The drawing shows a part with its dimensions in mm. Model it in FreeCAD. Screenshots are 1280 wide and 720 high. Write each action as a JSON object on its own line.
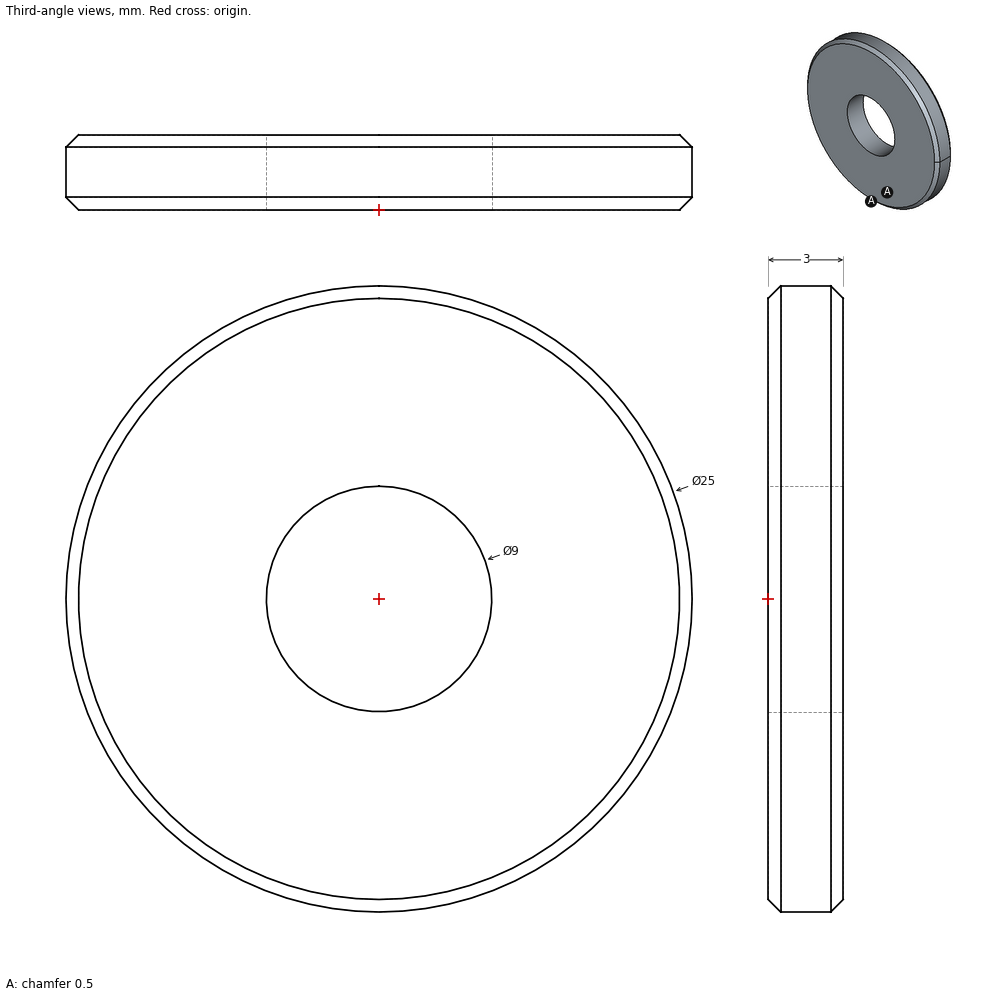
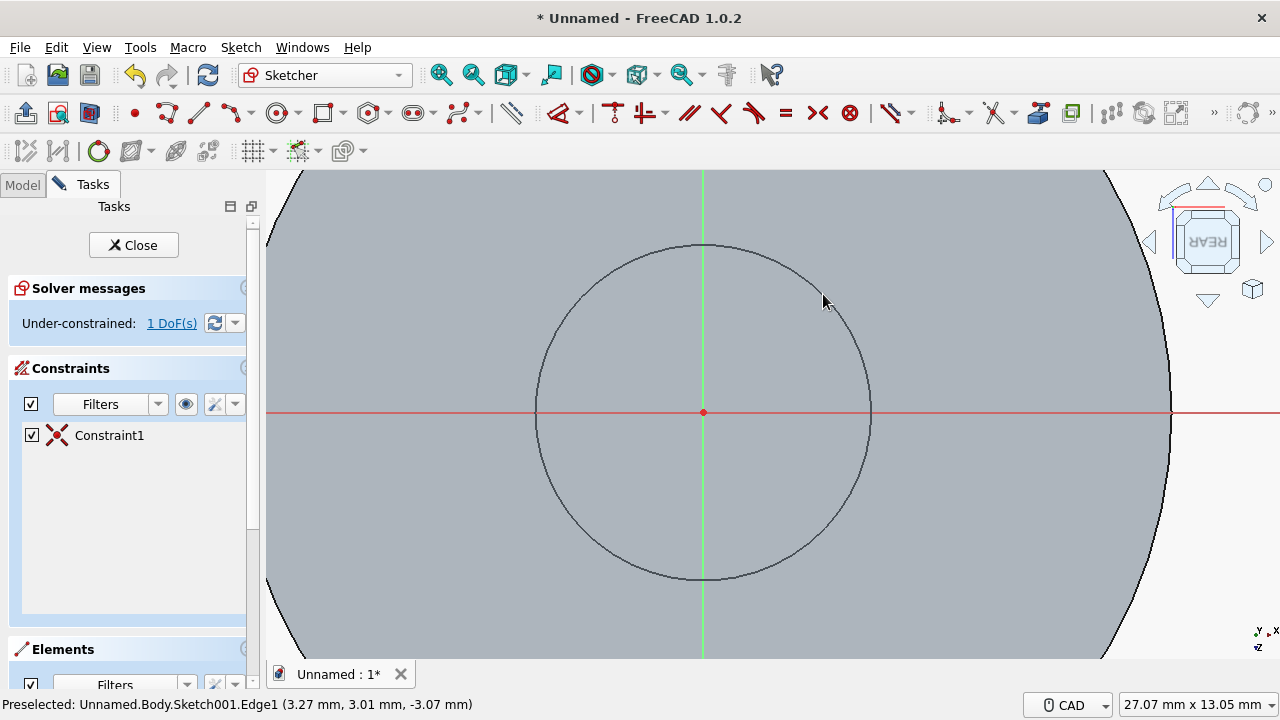
{"action": "left_click", "coordinate": [558, 114]}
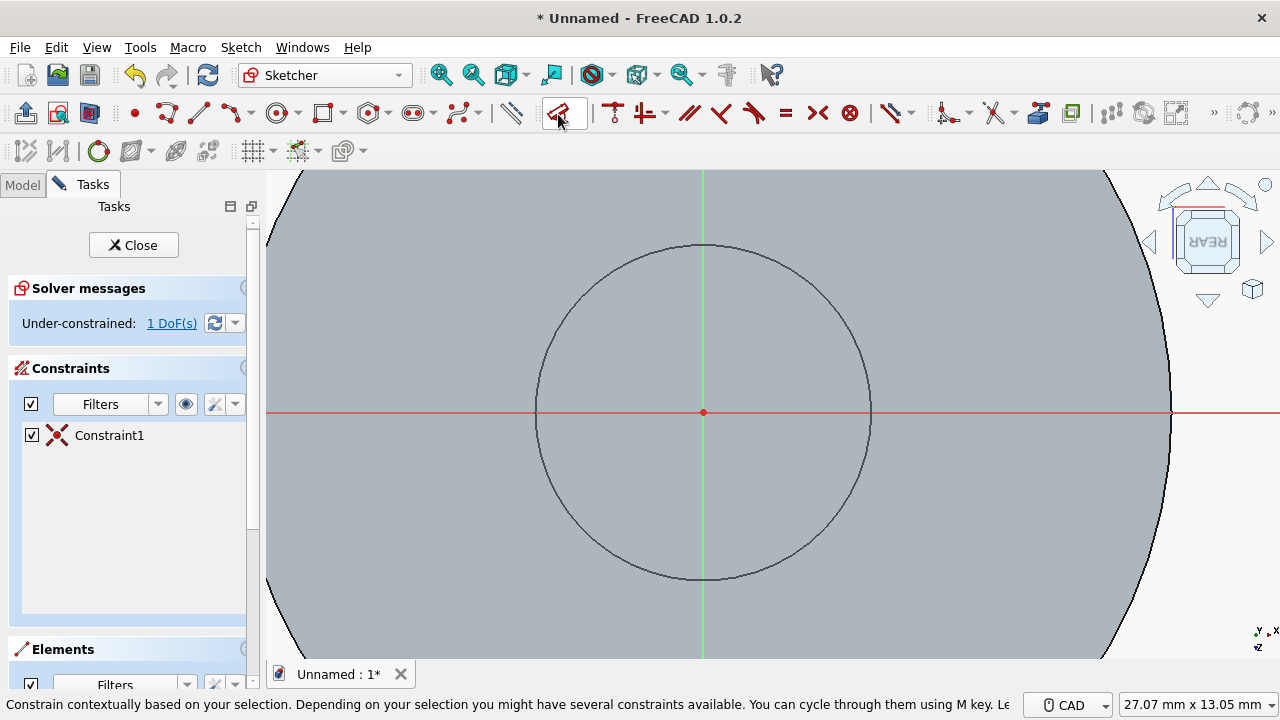
{"action": "left_click", "coordinate": [822, 294]}
{"action": "left_click", "coordinate": [845, 271]}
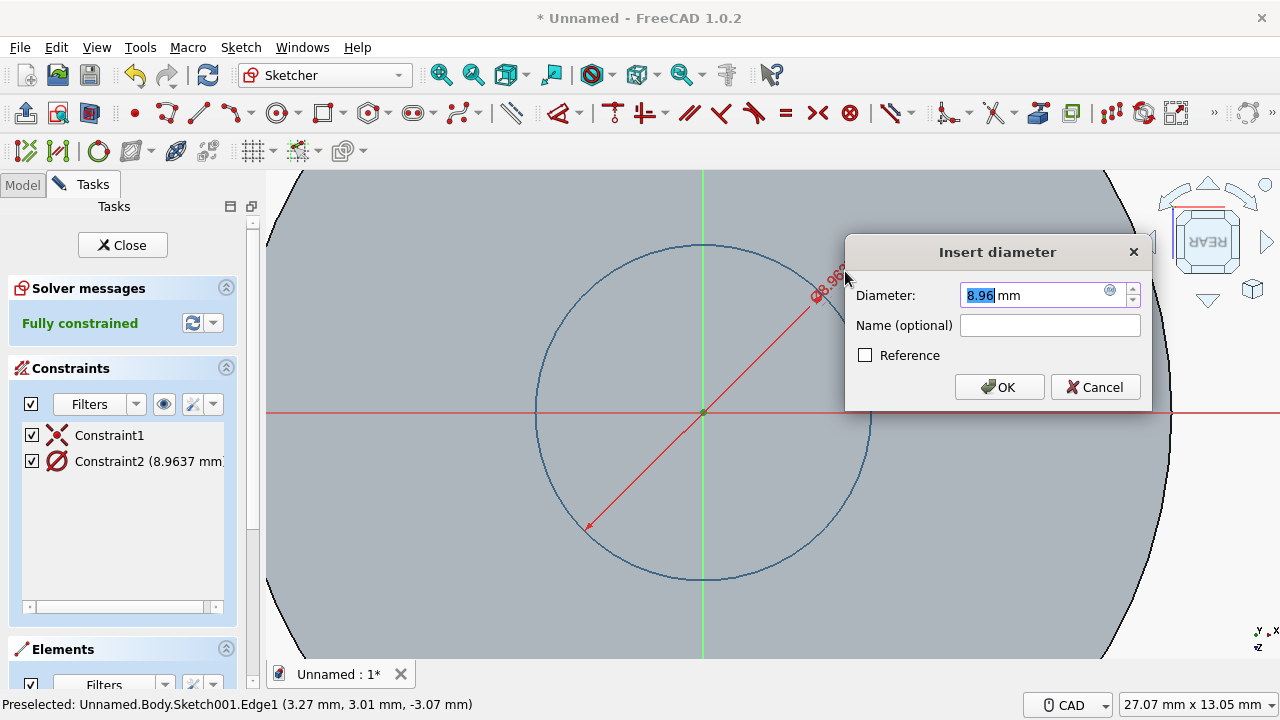
{"action": "type", "text": "9"}
{"action": "key", "text": "Return"}
{"action": "key", "text": "Escape"}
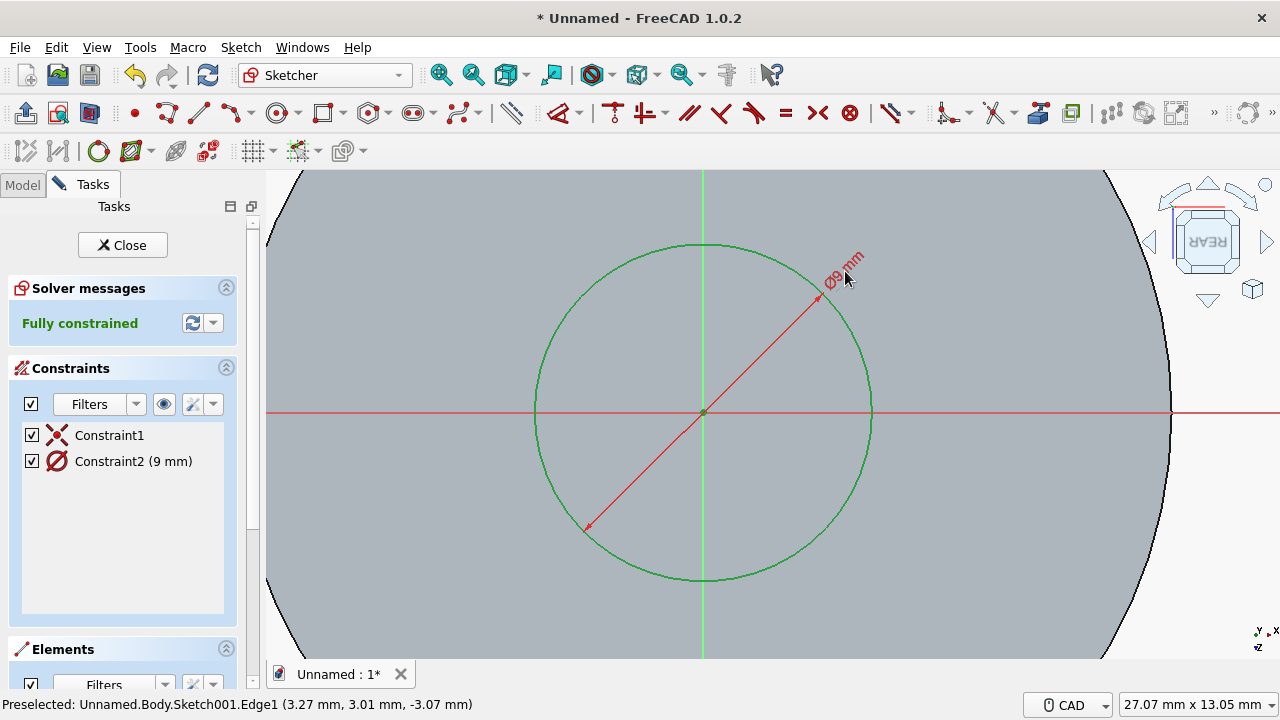
{"action": "left_click", "coordinate": [123, 245]}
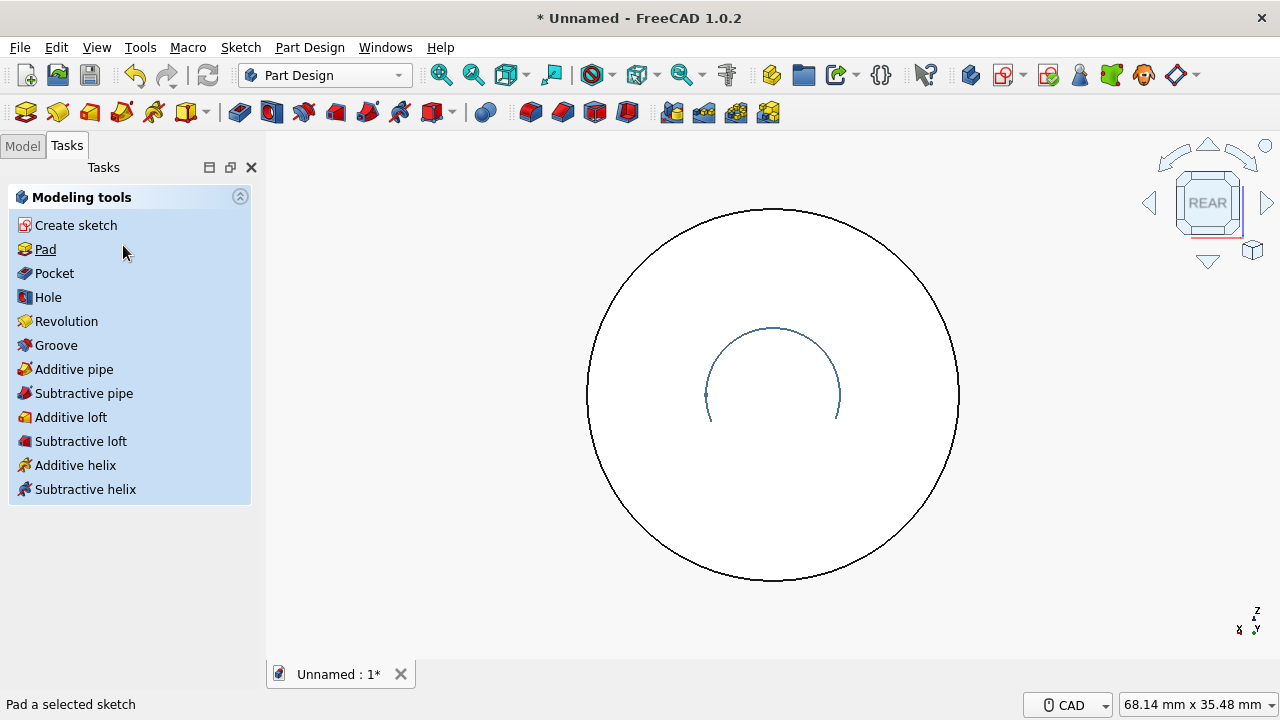
{"action": "left_click", "coordinate": [240, 112]}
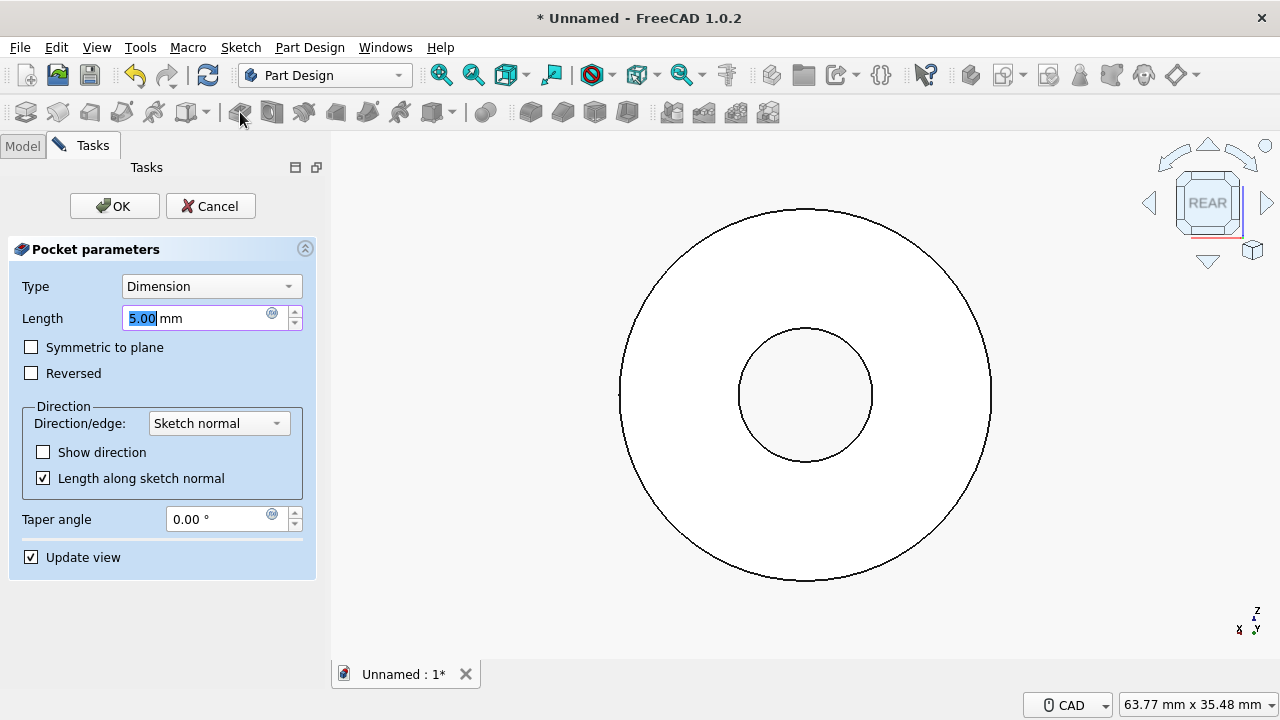
{"action": "left_click", "coordinate": [212, 286]}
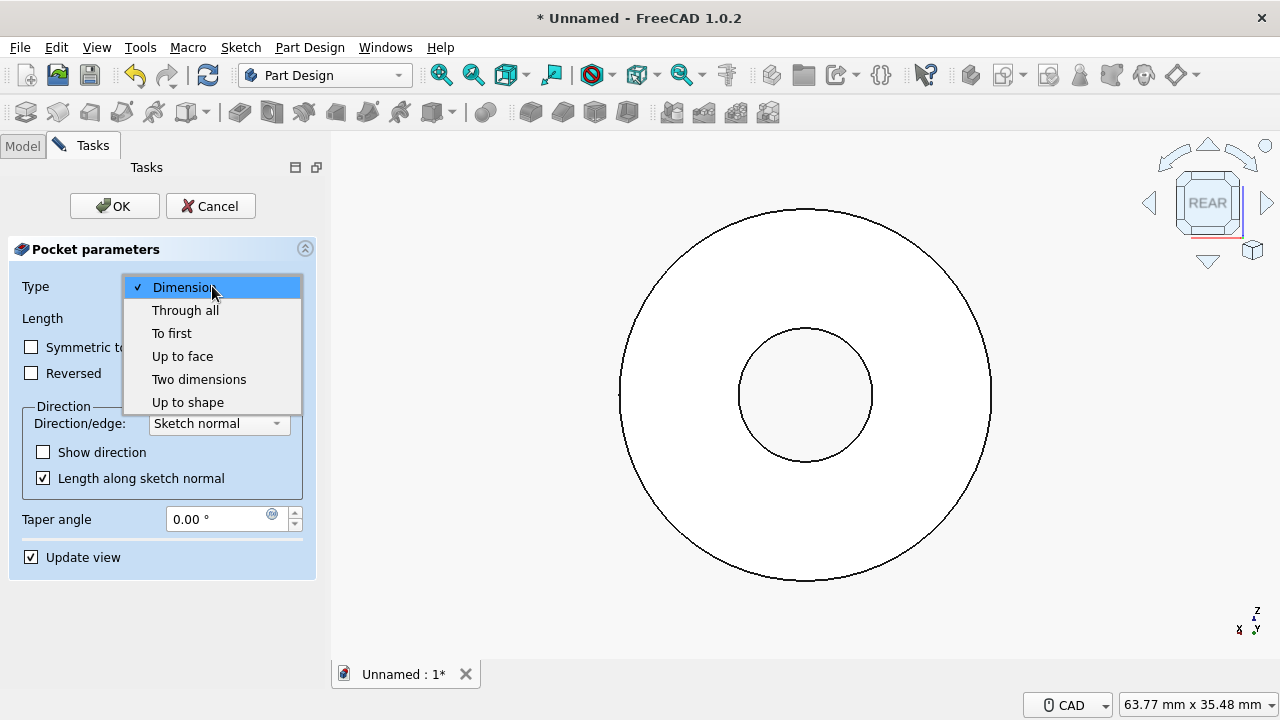
{"action": "left_click", "coordinate": [212, 310]}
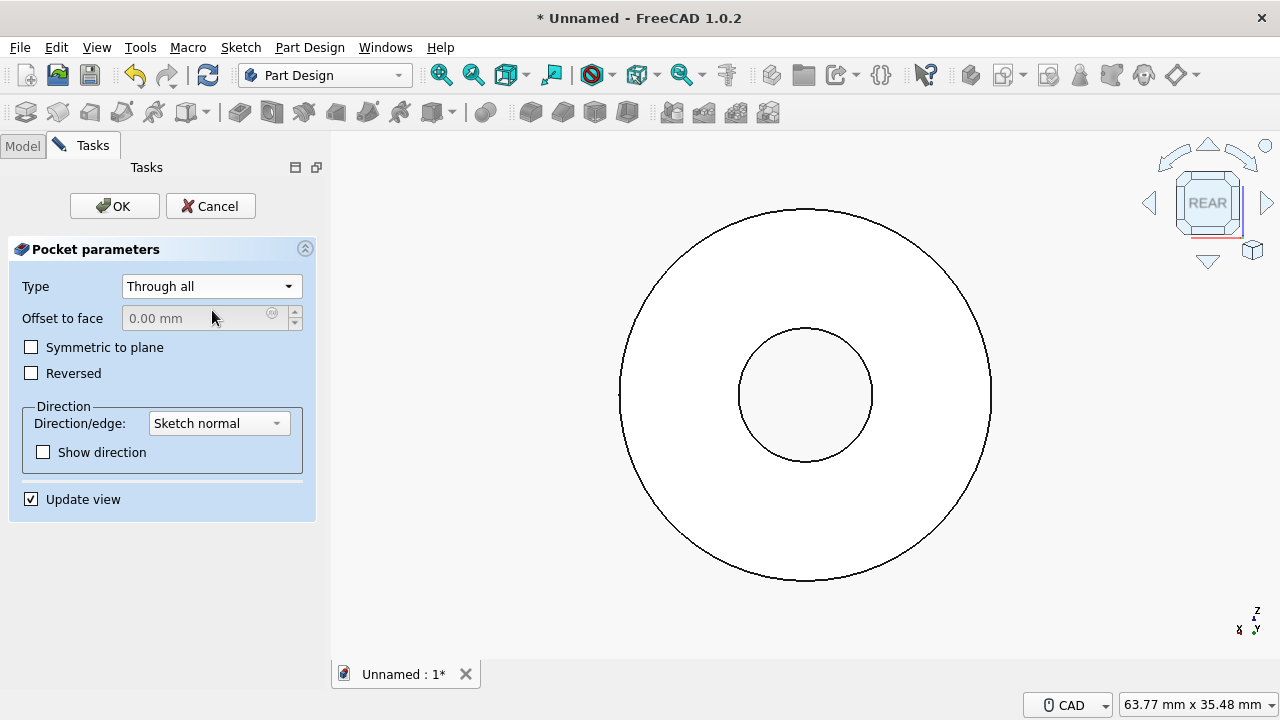
{"action": "left_click", "coordinate": [115, 206]}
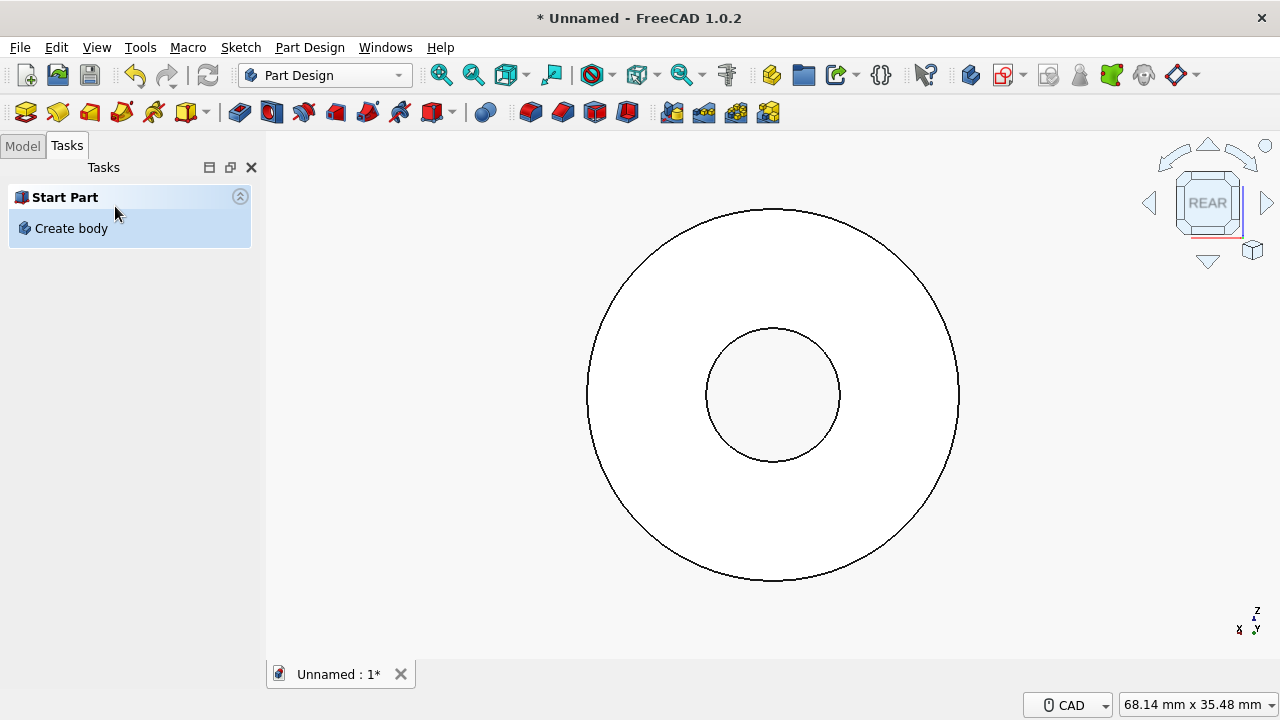
{"action": "left_click", "coordinate": [959, 394]}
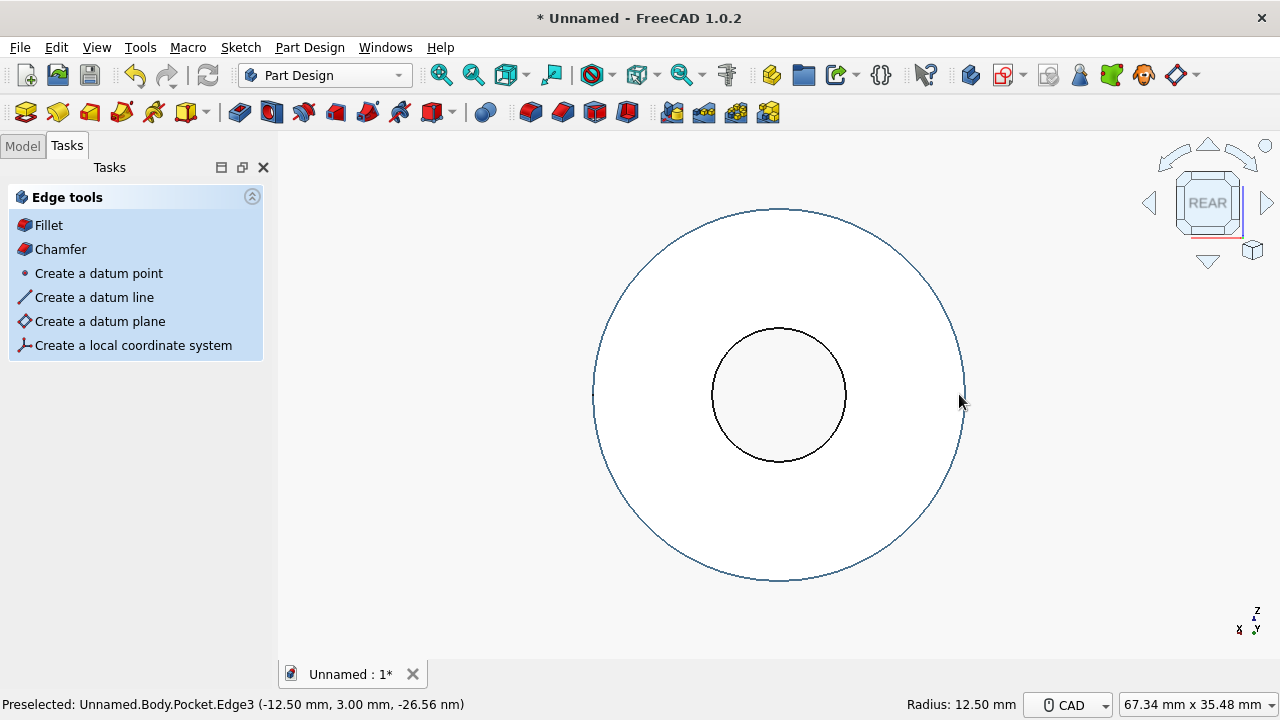
{"action": "key", "text": "0"}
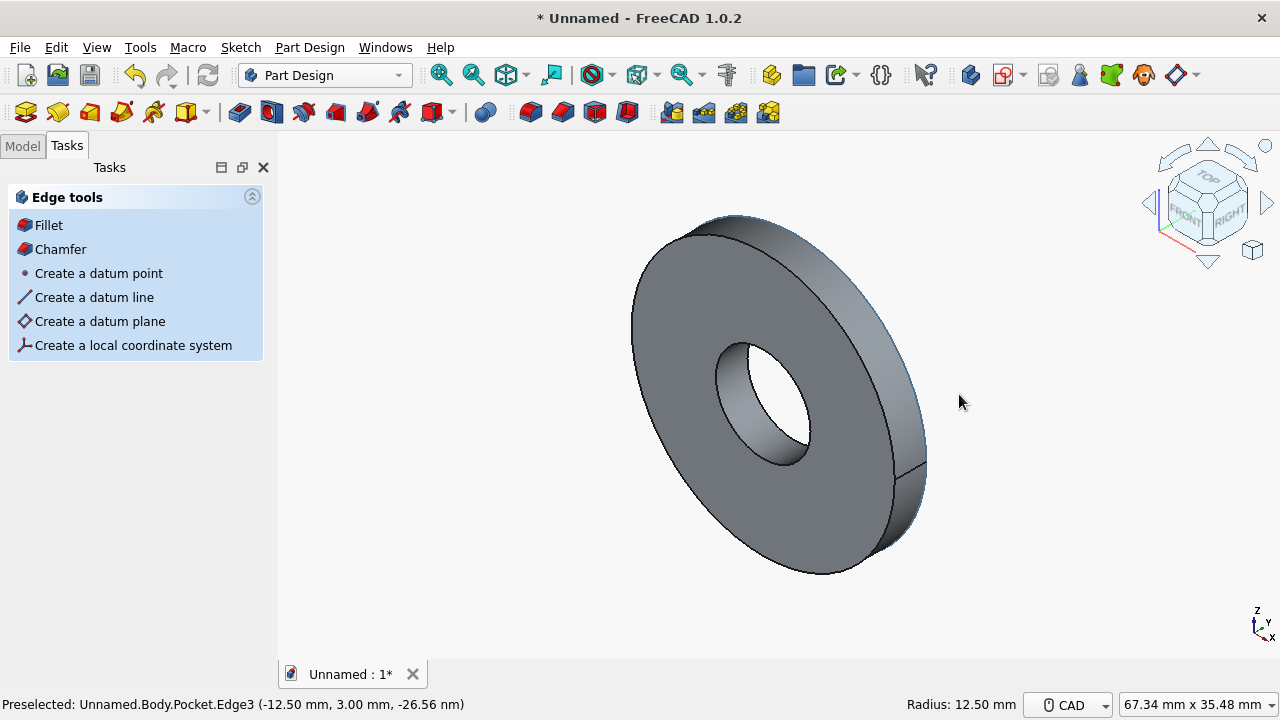
{"action": "left_click", "coordinate": [723, 235], "text": "ctrl"}